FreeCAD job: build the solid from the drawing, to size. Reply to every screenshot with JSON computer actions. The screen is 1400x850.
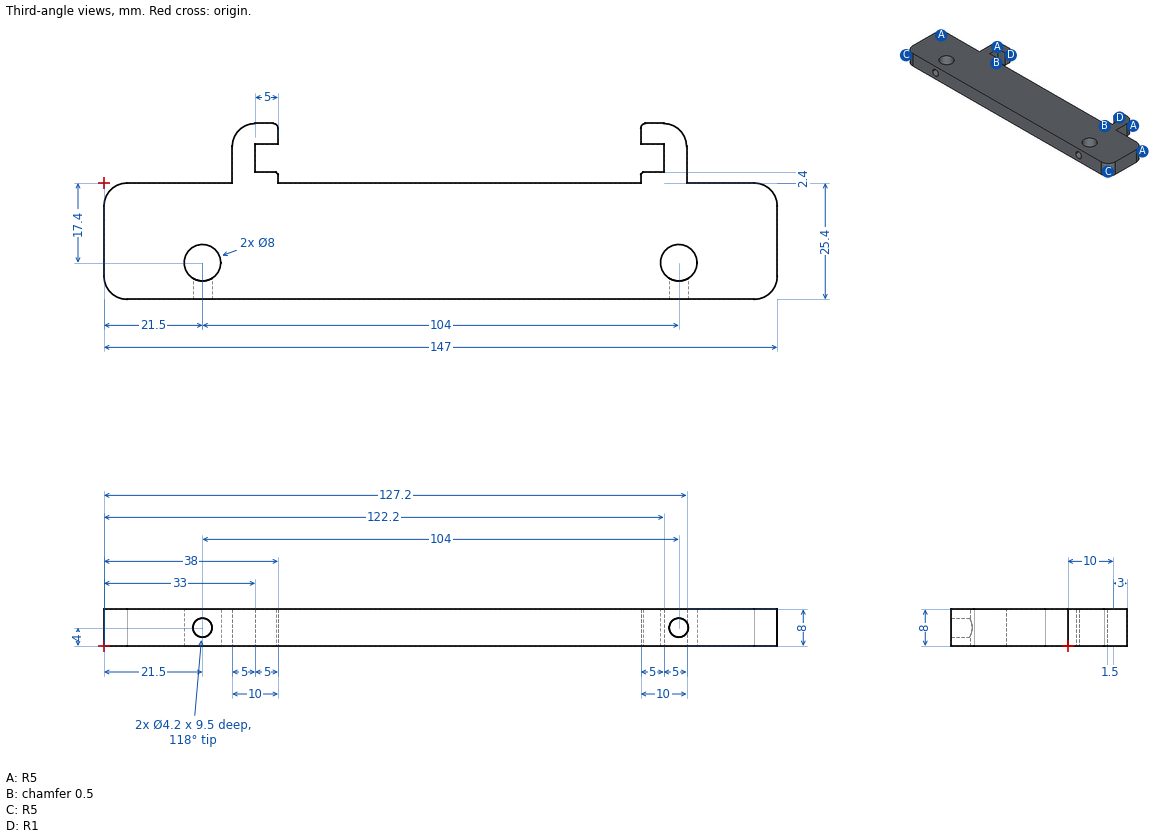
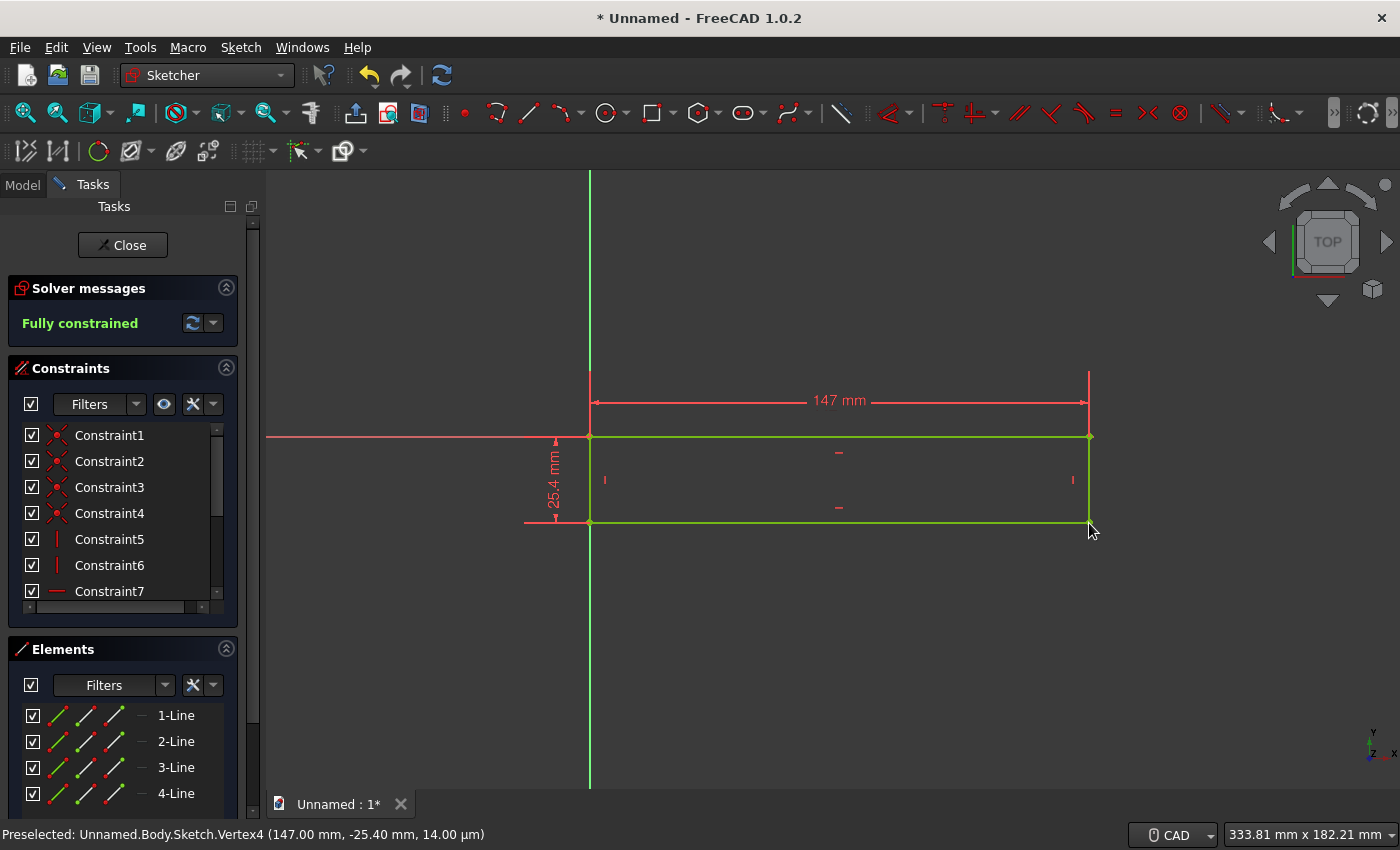
{"action": "left_click", "coordinate": [123, 245]}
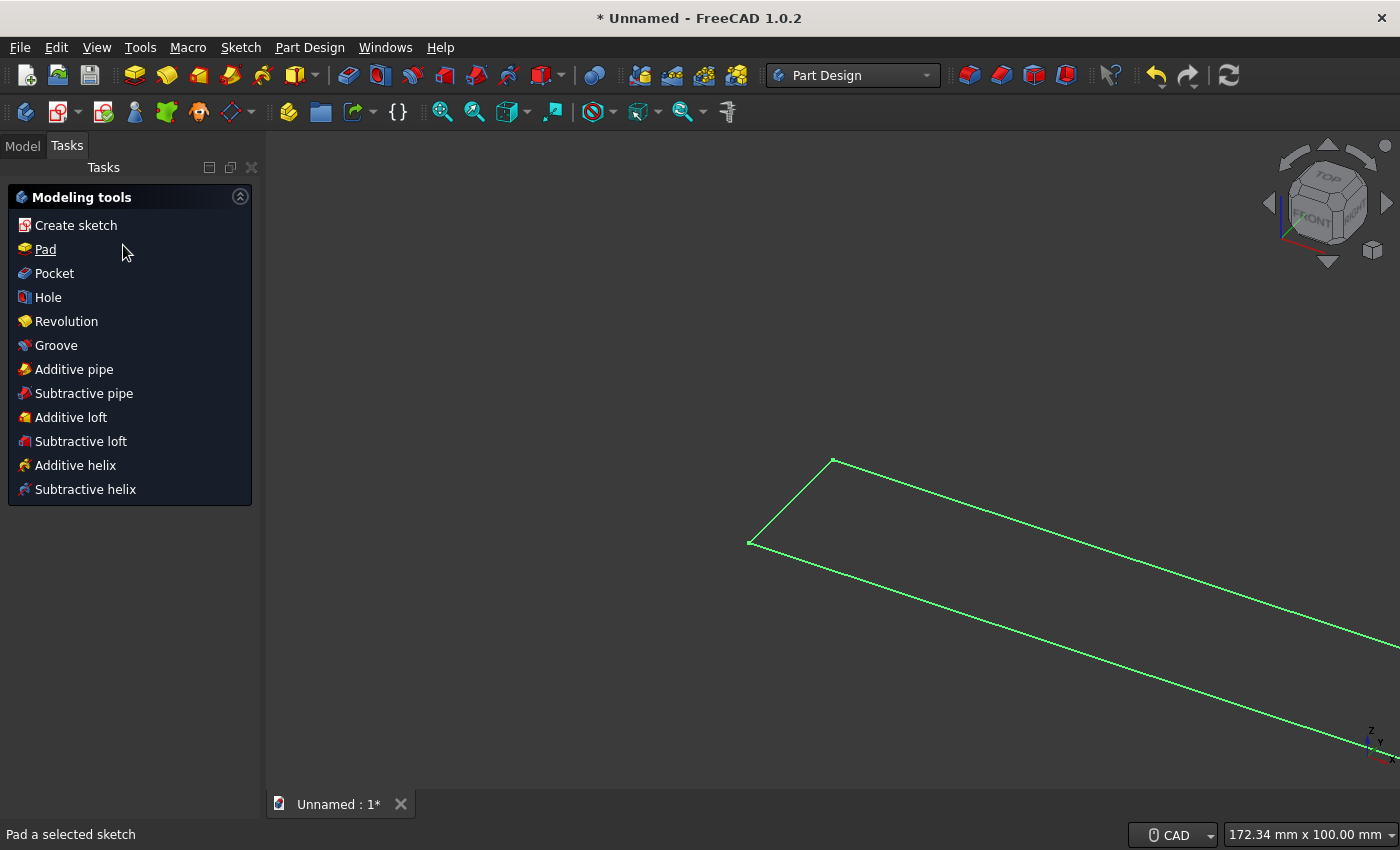
{"action": "left_click", "coordinate": [136, 76]}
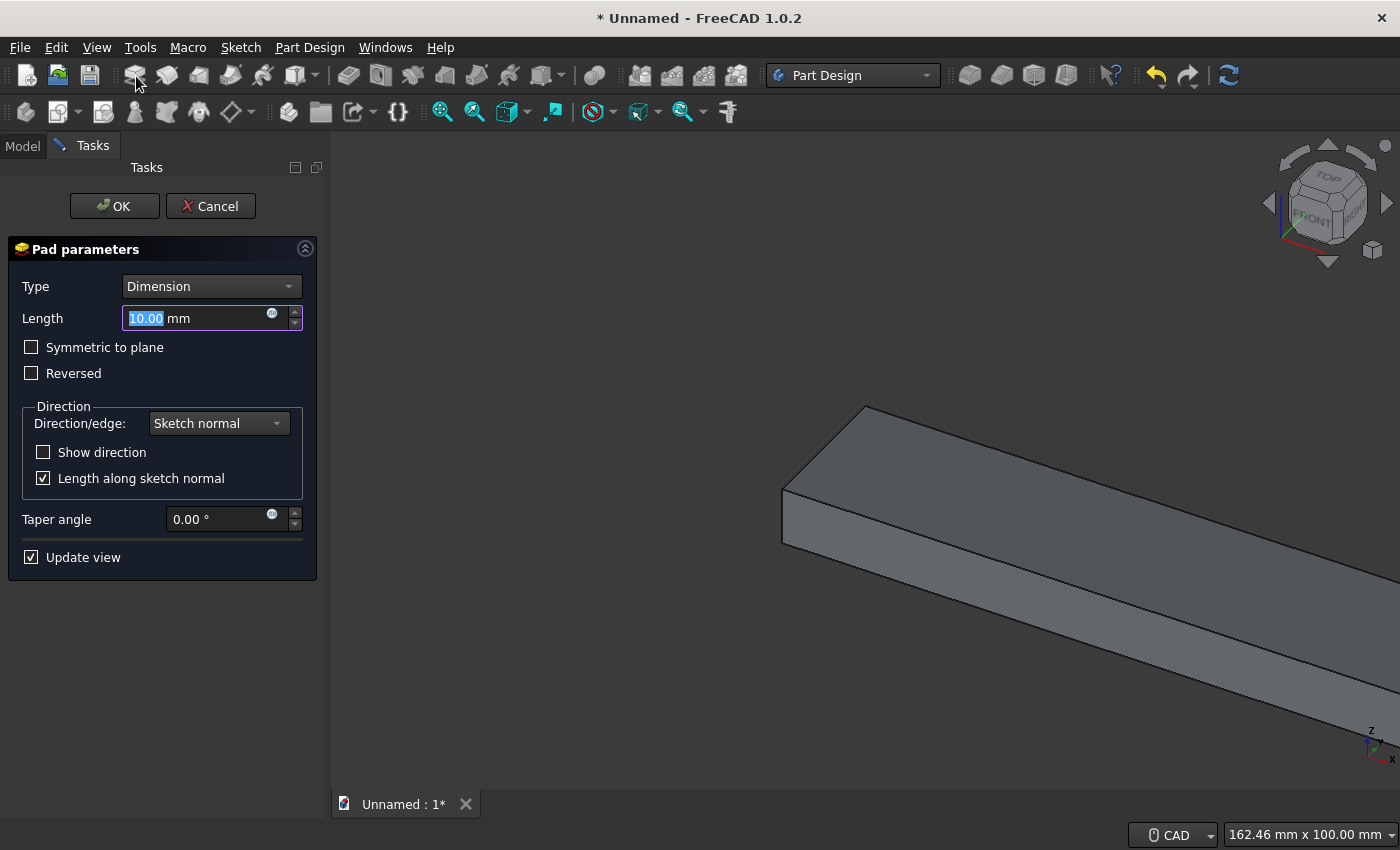
{"action": "type", "text": "8"}
{"action": "key", "text": "Tab"}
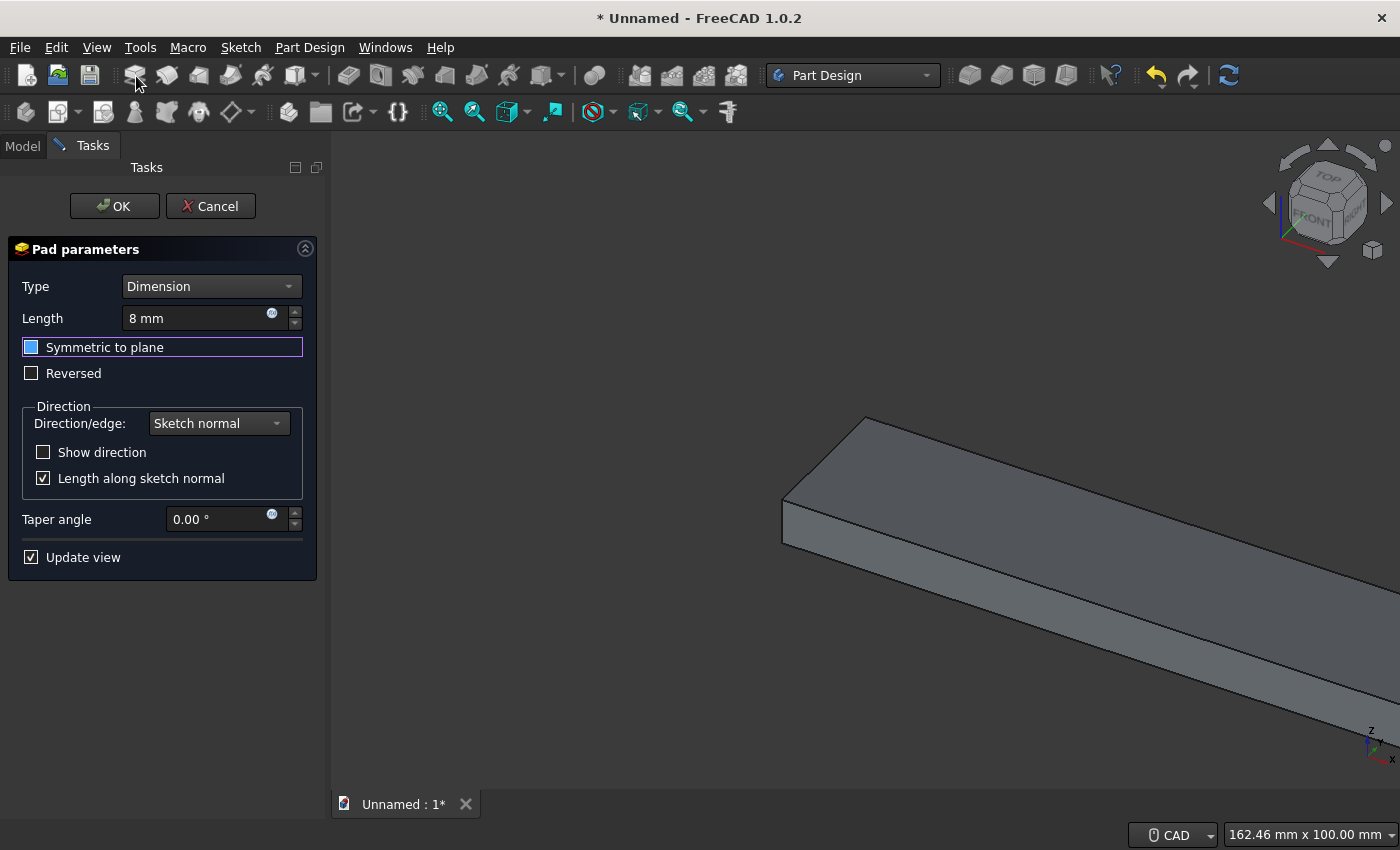
{"action": "left_click", "coordinate": [115, 206]}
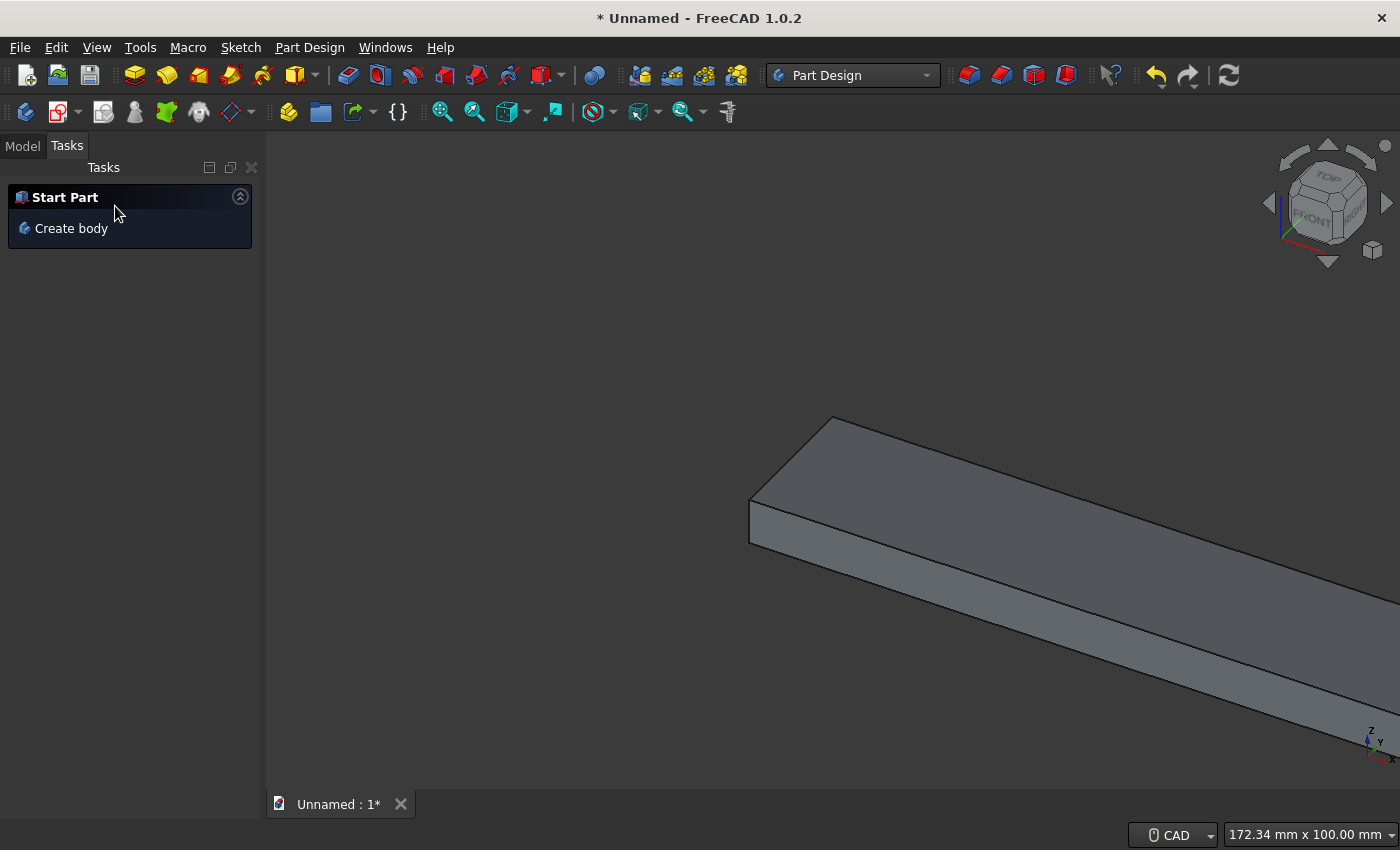
{"action": "left_click", "coordinate": [444, 112]}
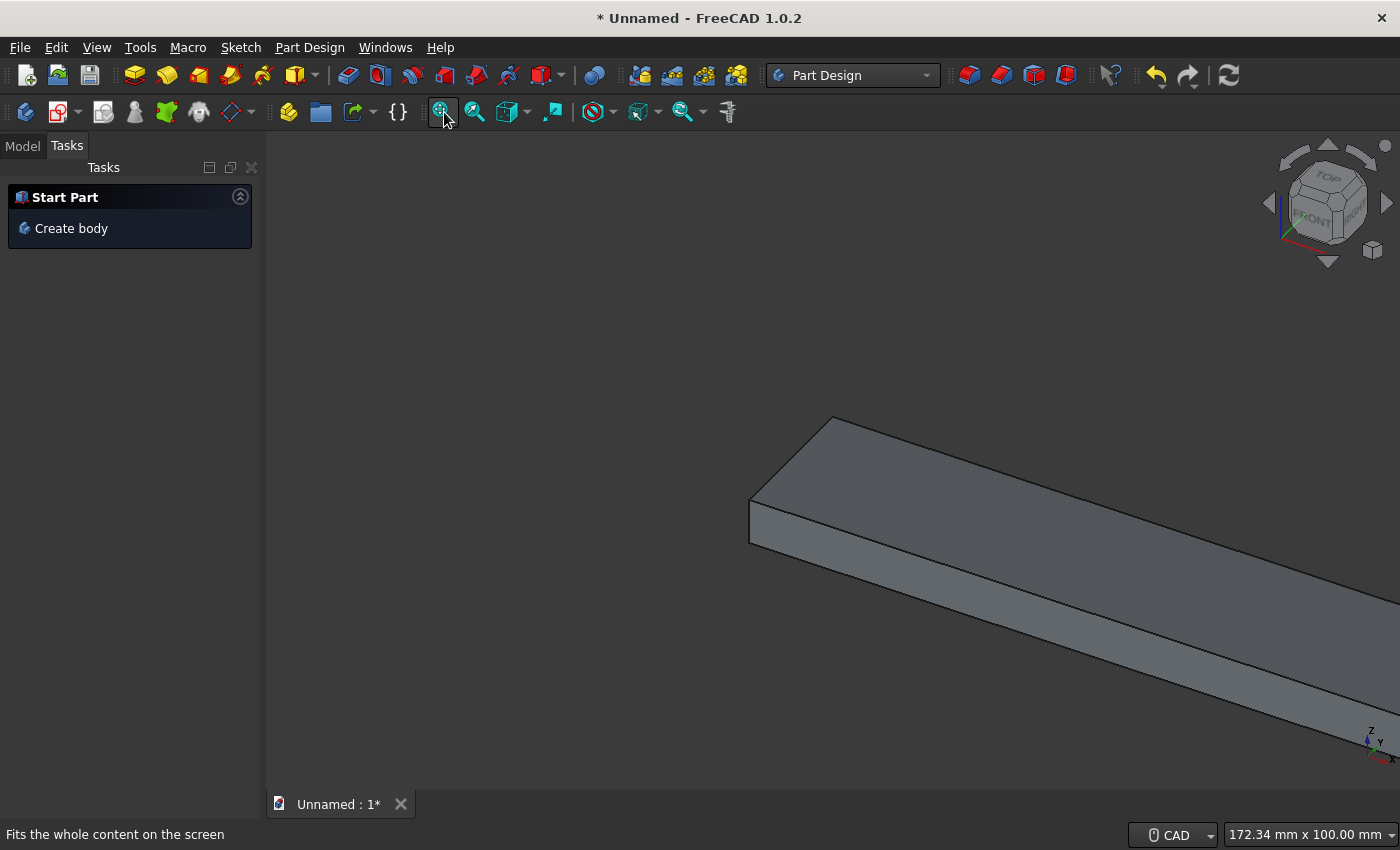
{"action": "key", "text": "4"}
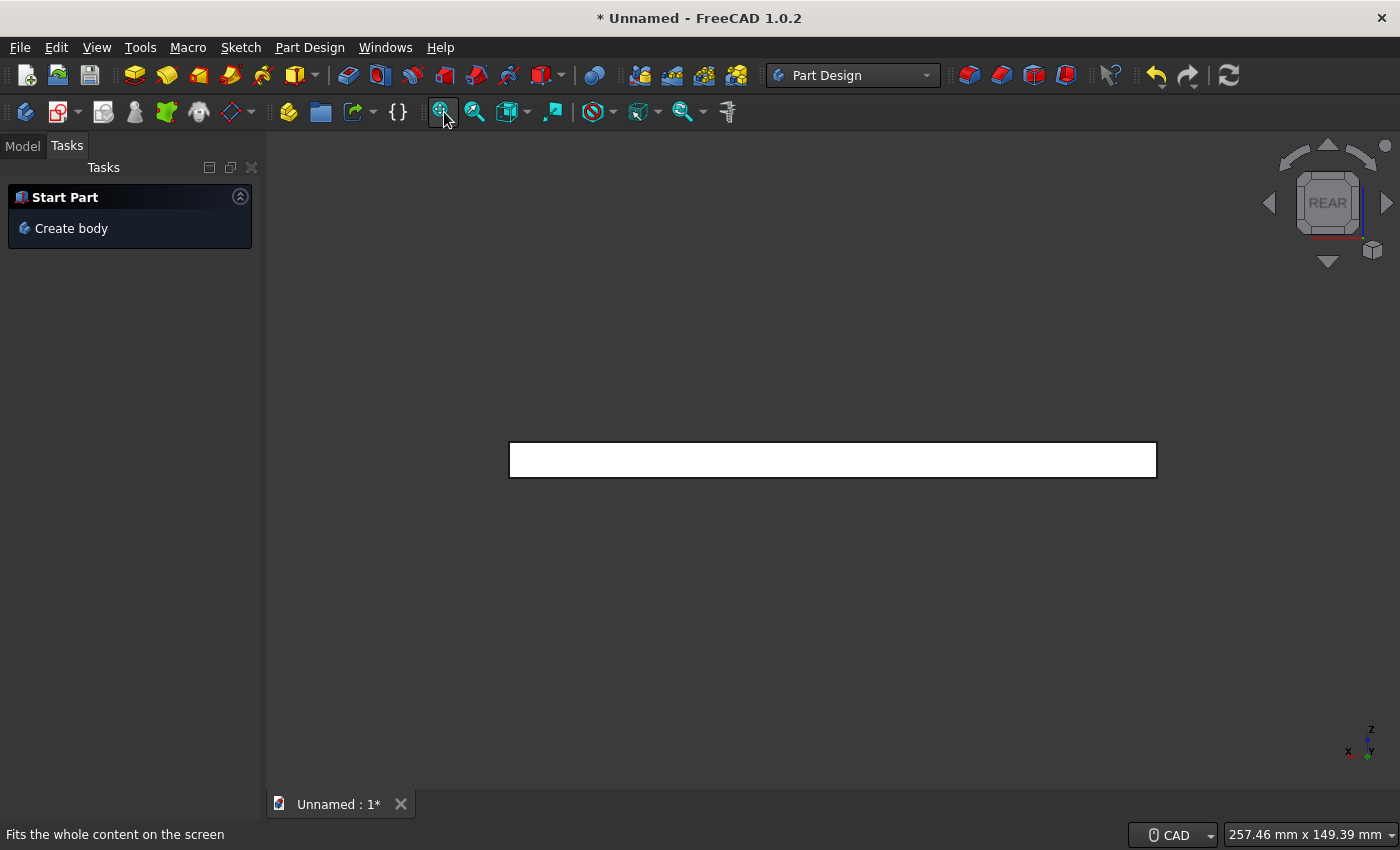
{"action": "left_click", "coordinate": [556, 459]}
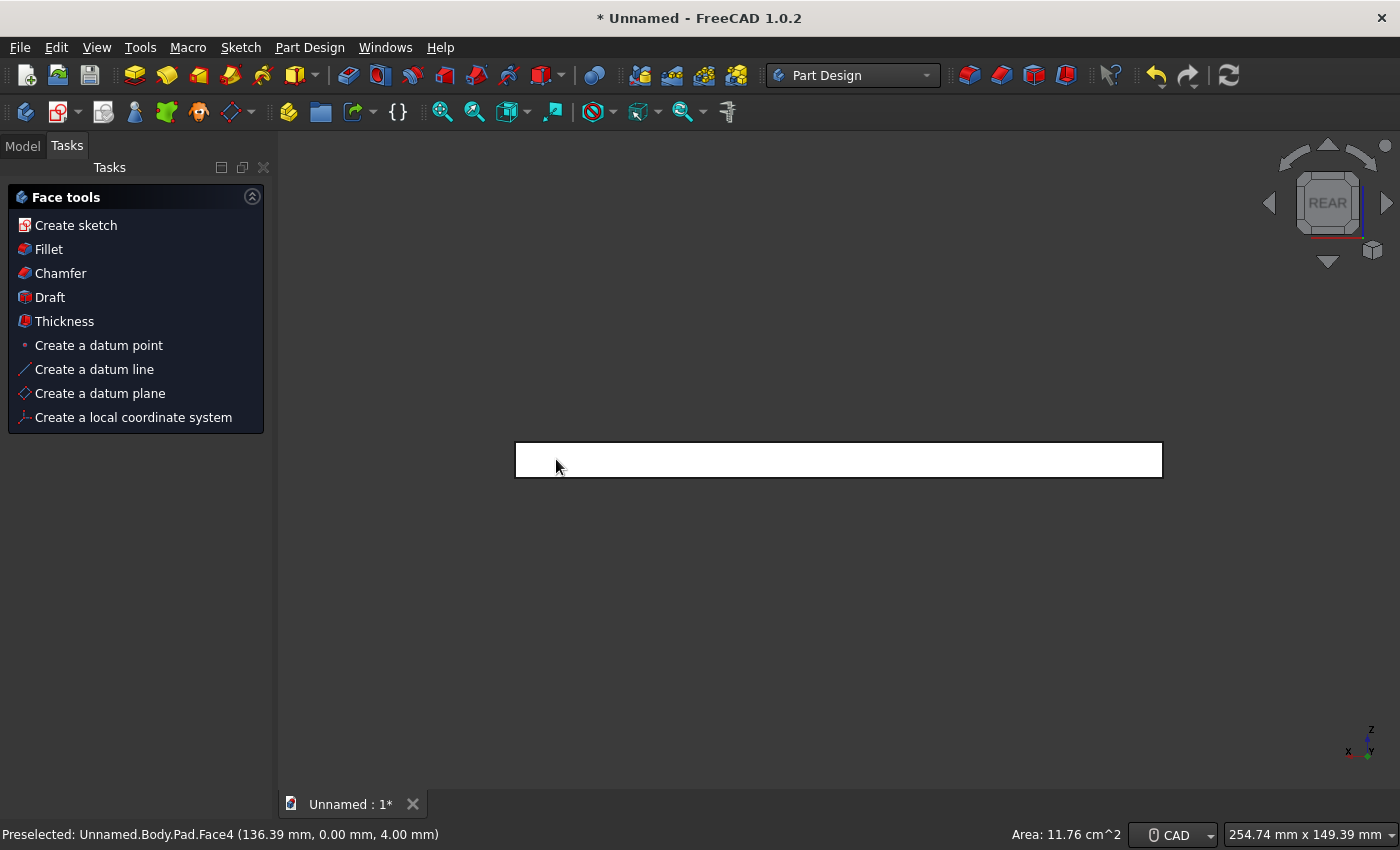
{"action": "left_click", "coordinate": [58, 112]}